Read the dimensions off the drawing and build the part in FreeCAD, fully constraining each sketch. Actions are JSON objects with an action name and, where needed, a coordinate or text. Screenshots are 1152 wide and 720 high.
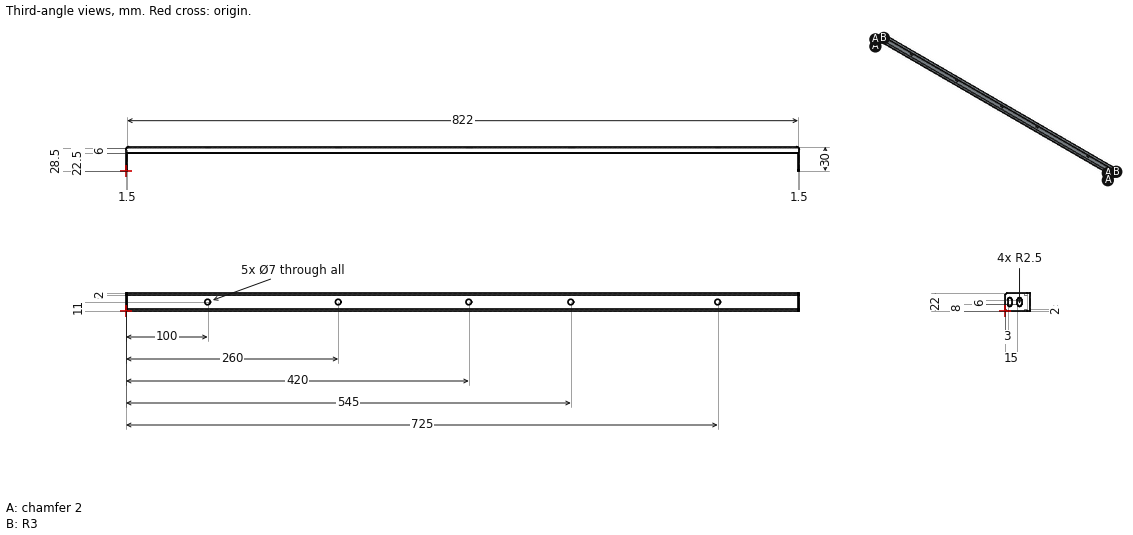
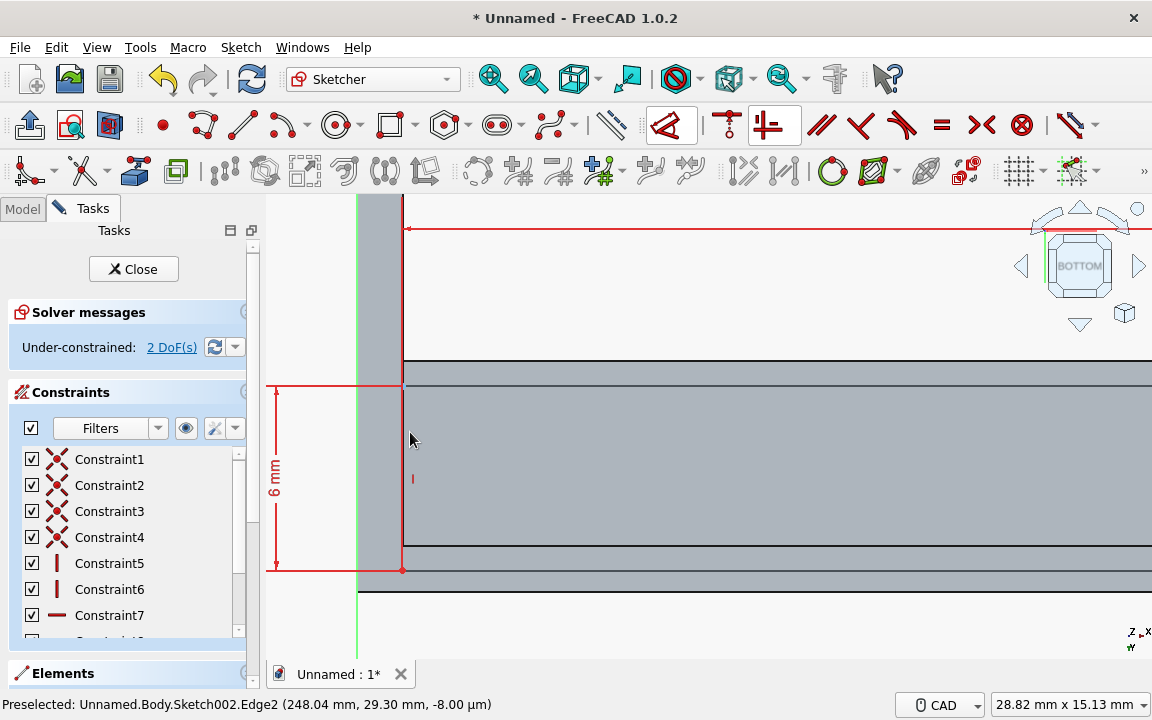
{"action": "left_click", "coordinate": [402, 386]}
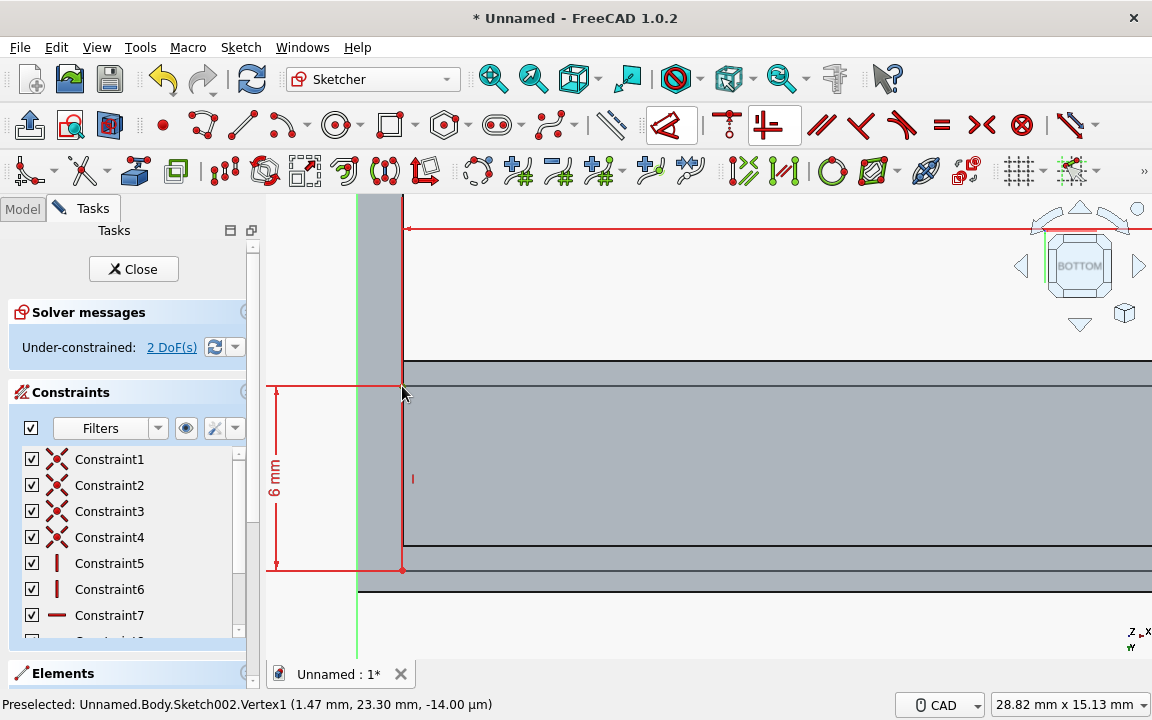
{"action": "left_click", "coordinate": [692, 126]}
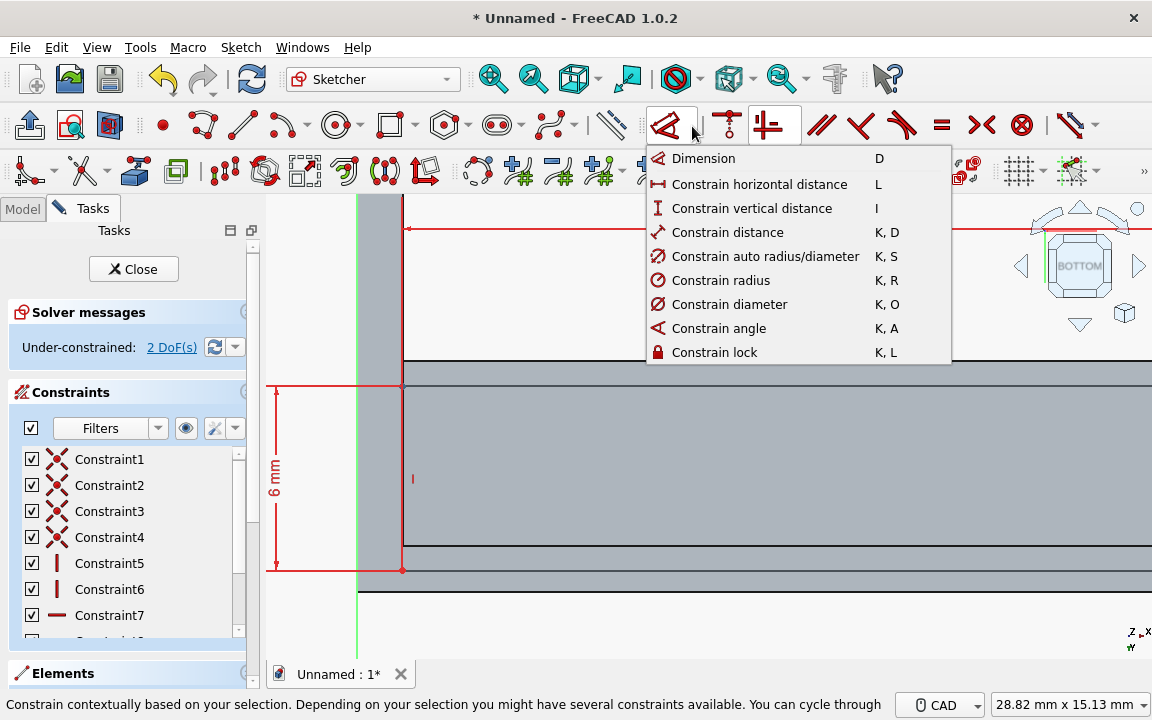
{"action": "left_click", "coordinate": [799, 184]}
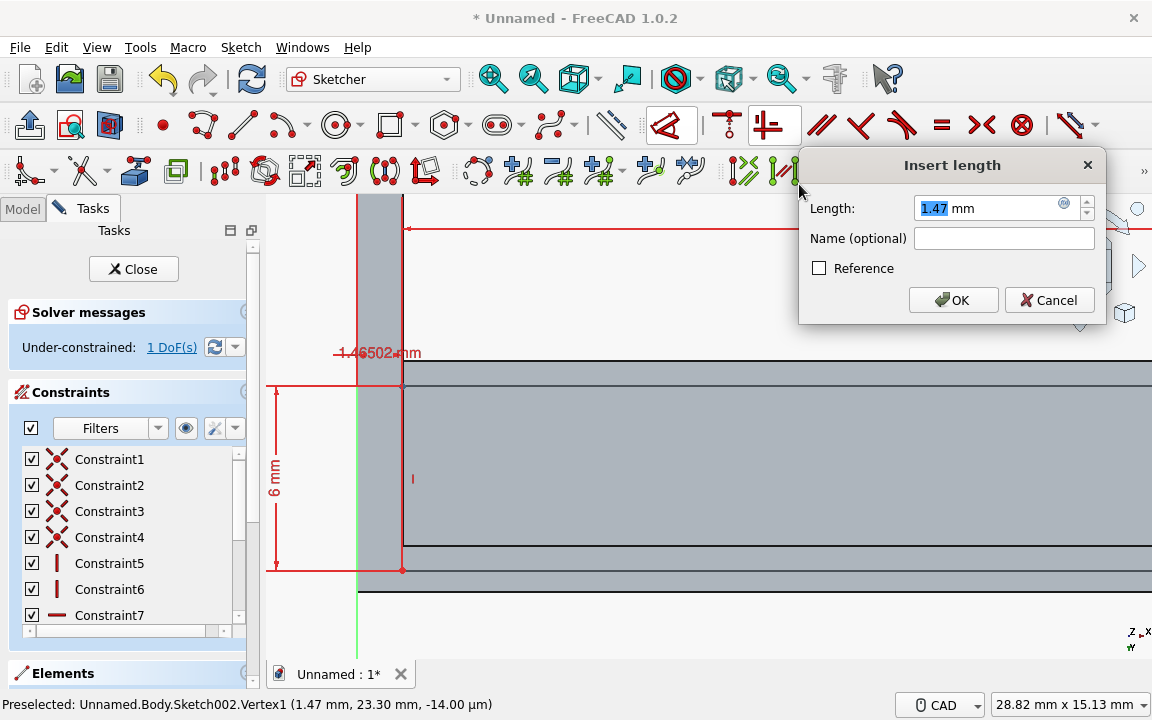
{"action": "type", "text": "1.5"}
{"action": "key", "text": "Return"}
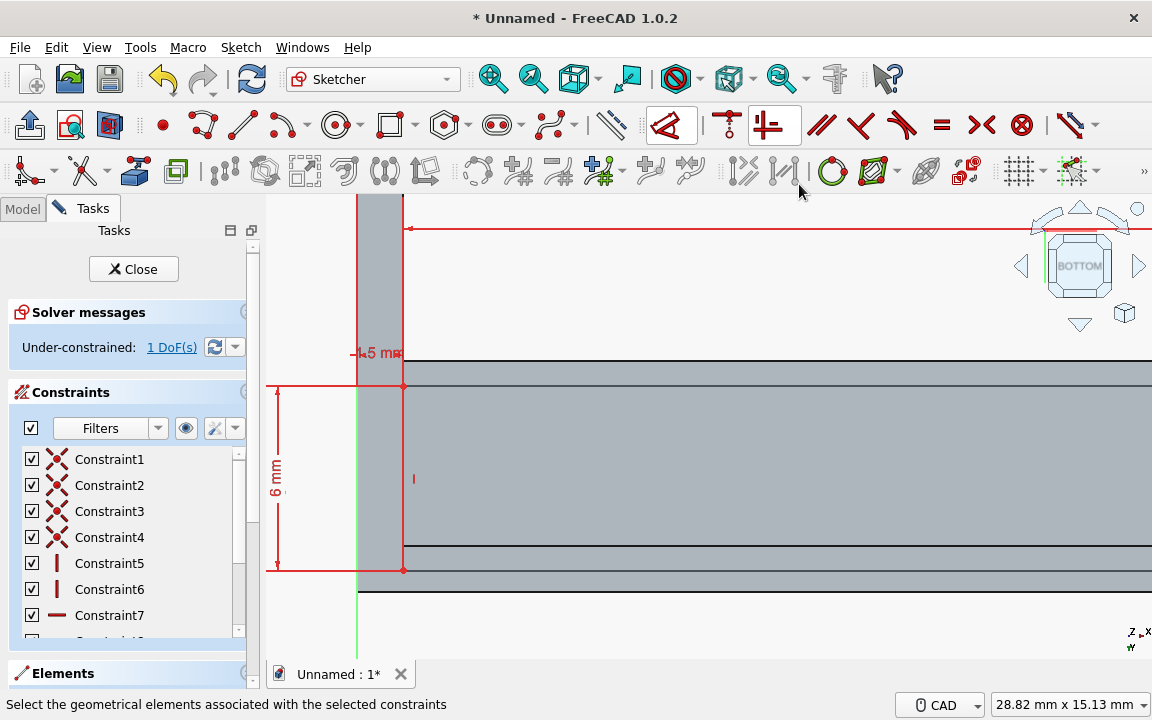
{"action": "scroll", "coordinate": [640, 426], "scroll_direction": "down", "scroll_amount": 15}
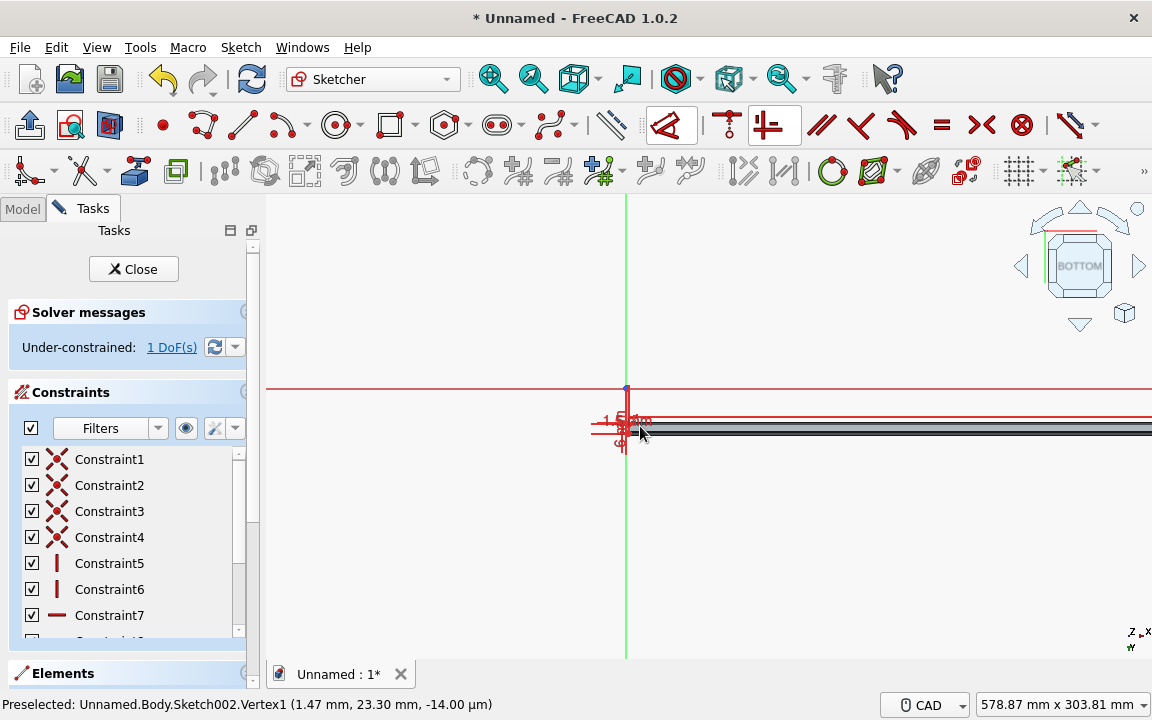
{"action": "scroll", "coordinate": [294, 436], "scroll_direction": "down", "scroll_amount": 5}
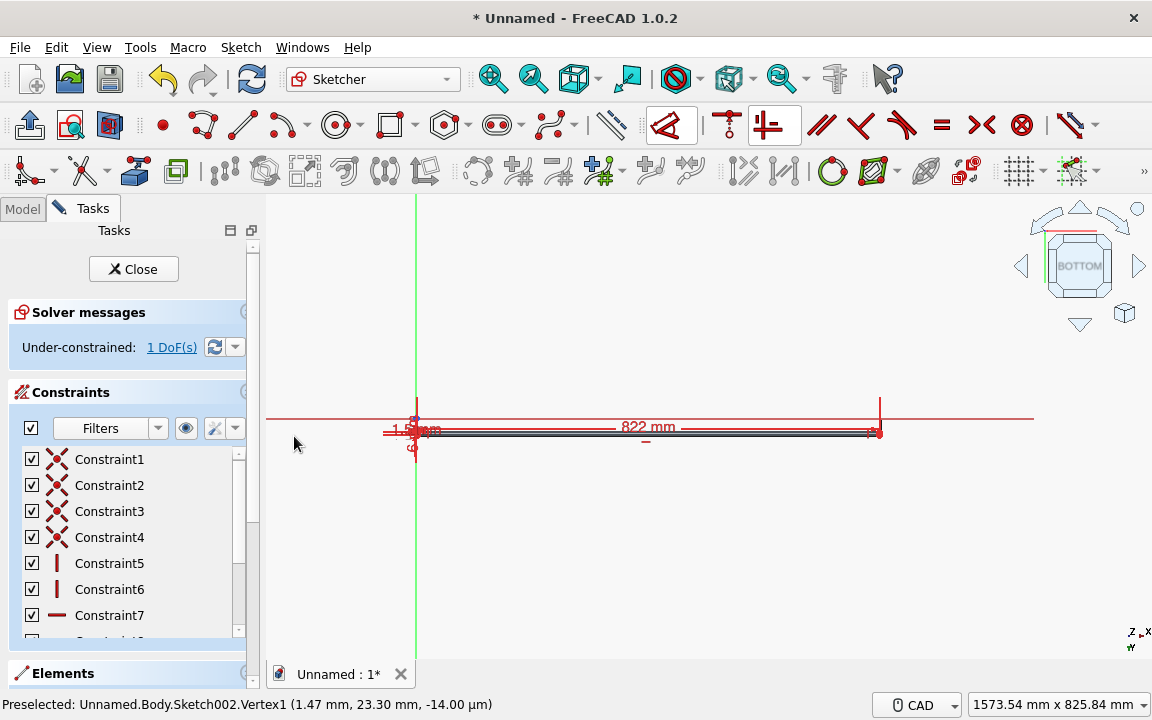
{"action": "scroll", "coordinate": [417, 432], "scroll_direction": "up", "scroll_amount": 7}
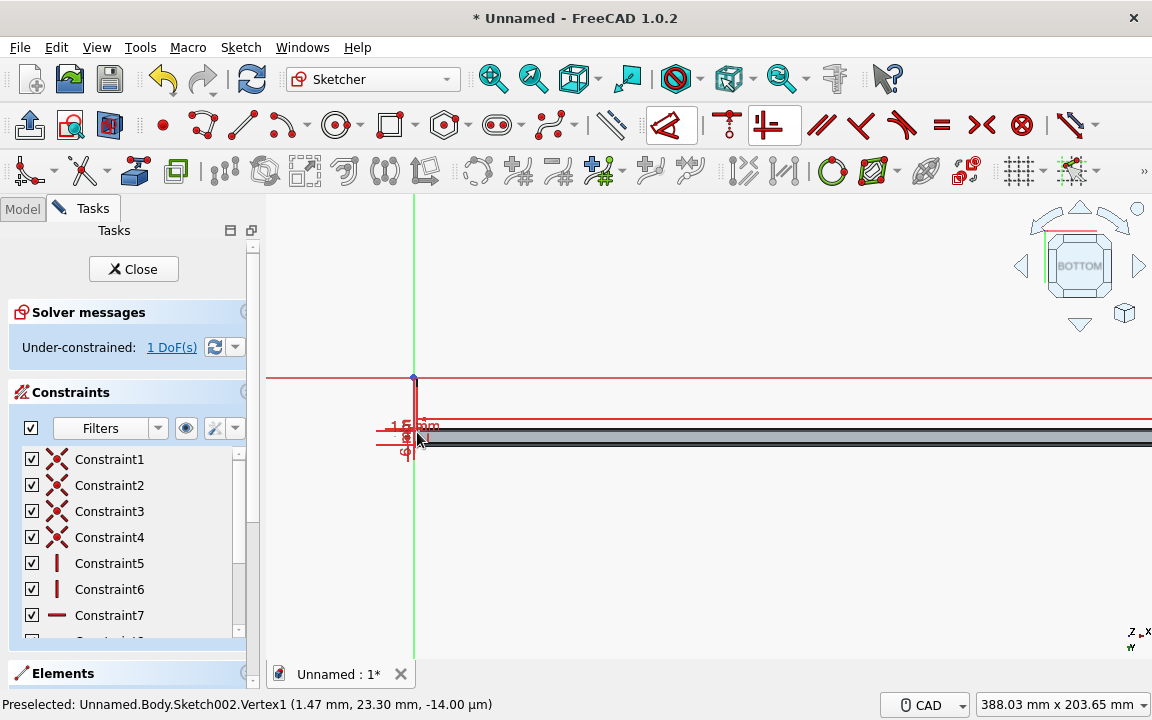
{"action": "left_click", "coordinate": [417, 431]}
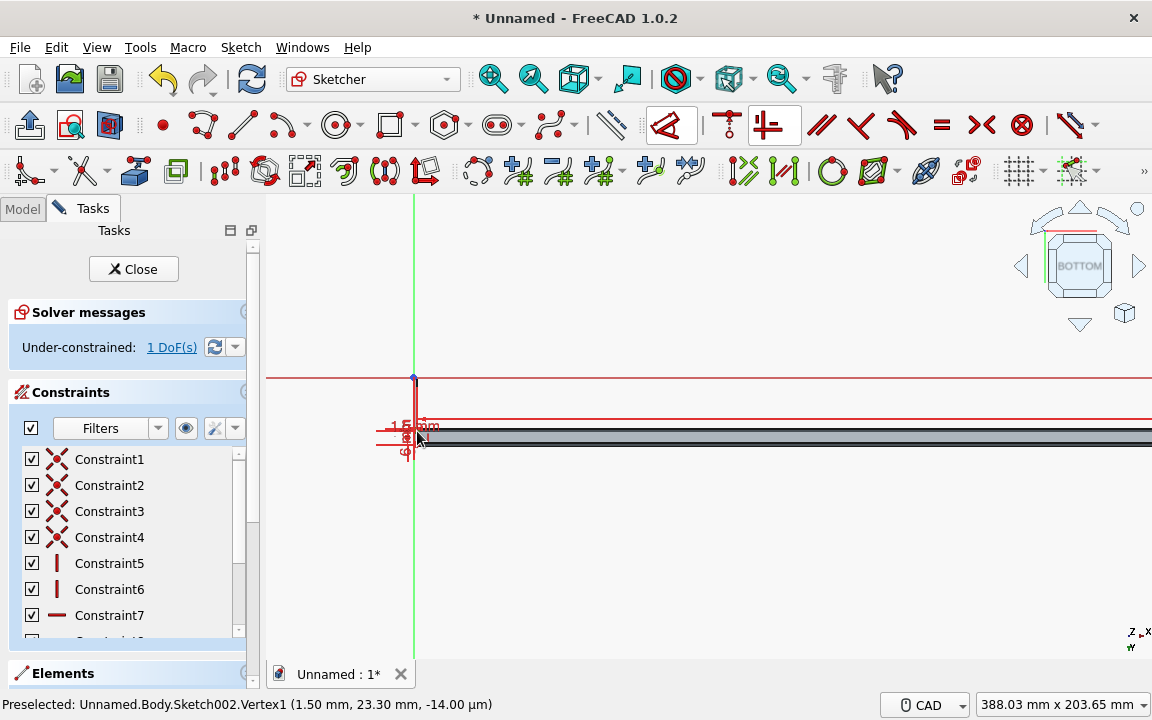
{"action": "key", "text": "i"}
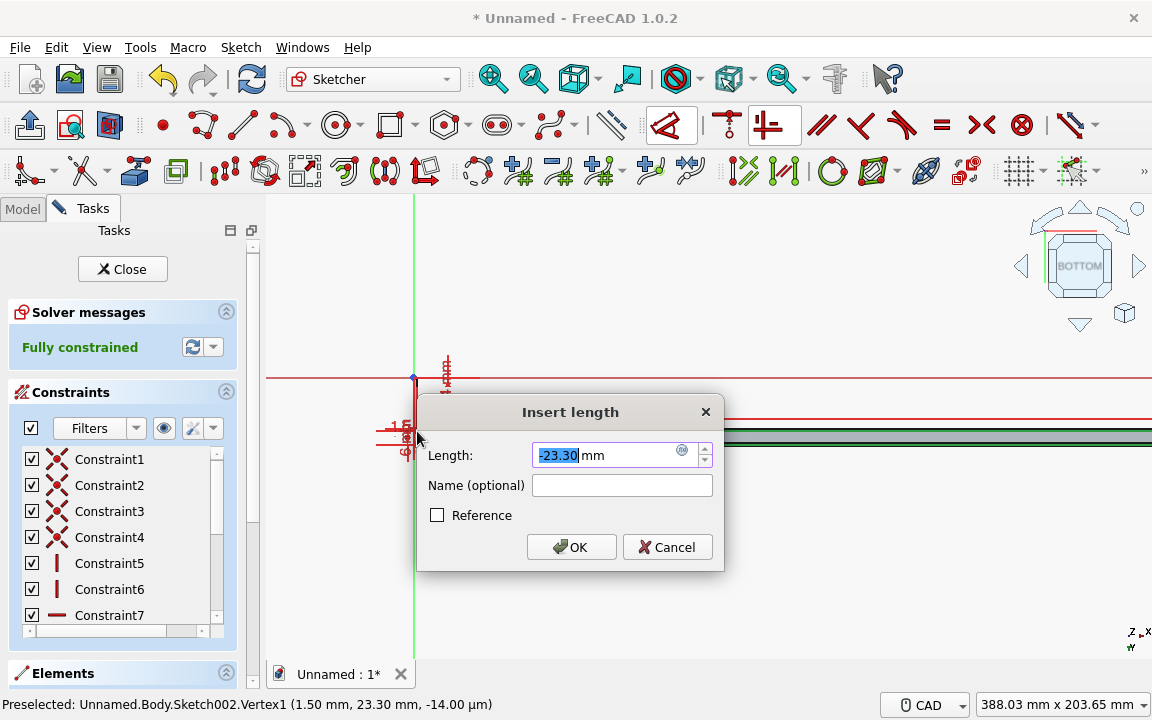
{"action": "type", "text": "-22.5"}
{"action": "key", "text": "Return"}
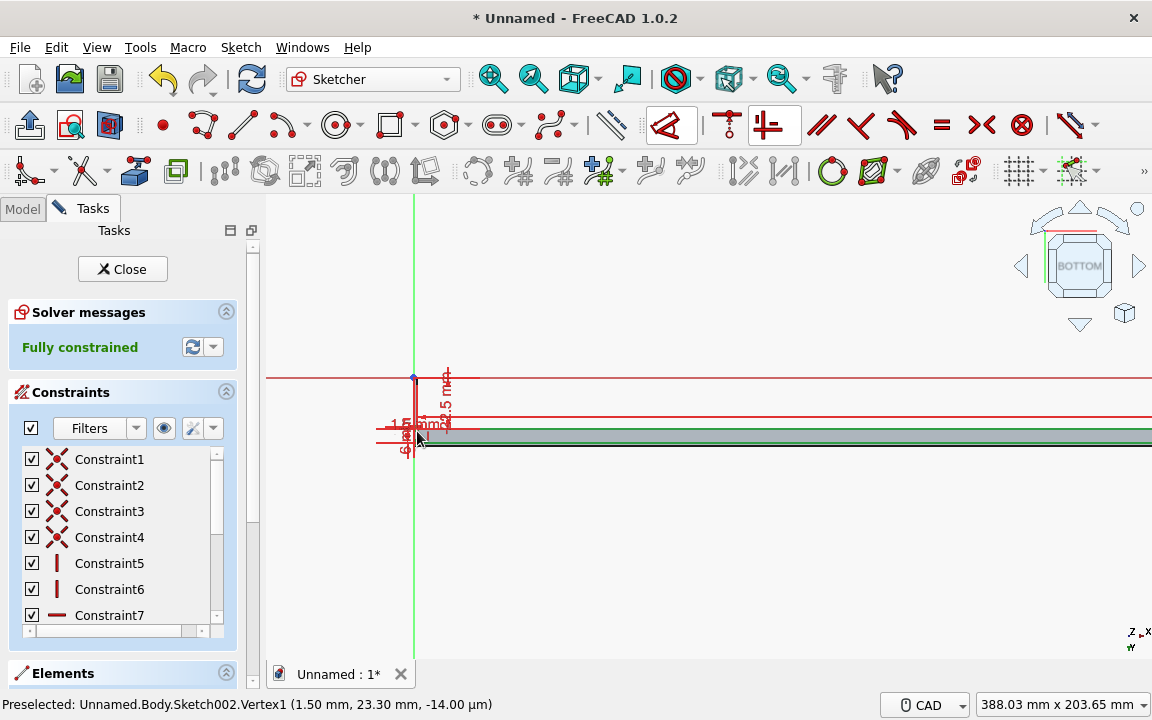
{"action": "left_click", "coordinate": [123, 269]}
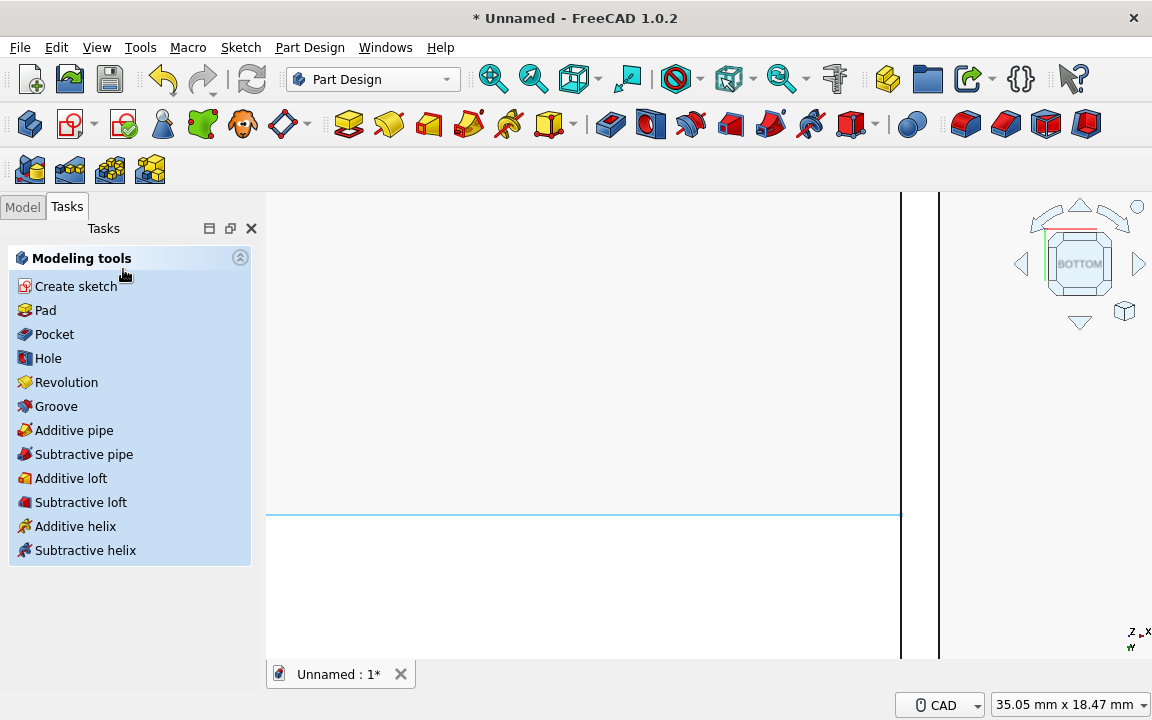
{"action": "left_click", "coordinate": [350, 124]}